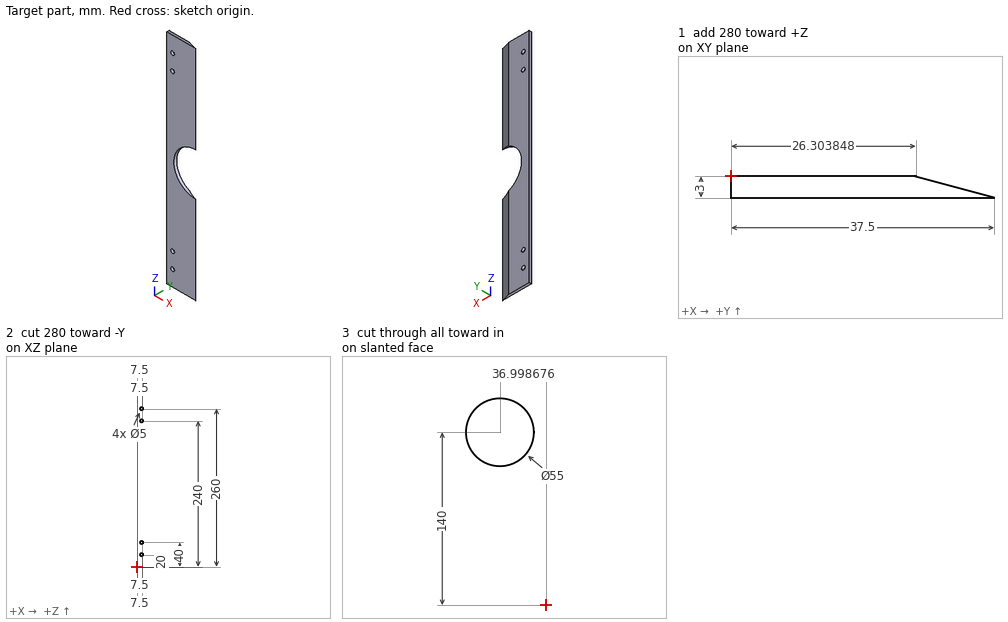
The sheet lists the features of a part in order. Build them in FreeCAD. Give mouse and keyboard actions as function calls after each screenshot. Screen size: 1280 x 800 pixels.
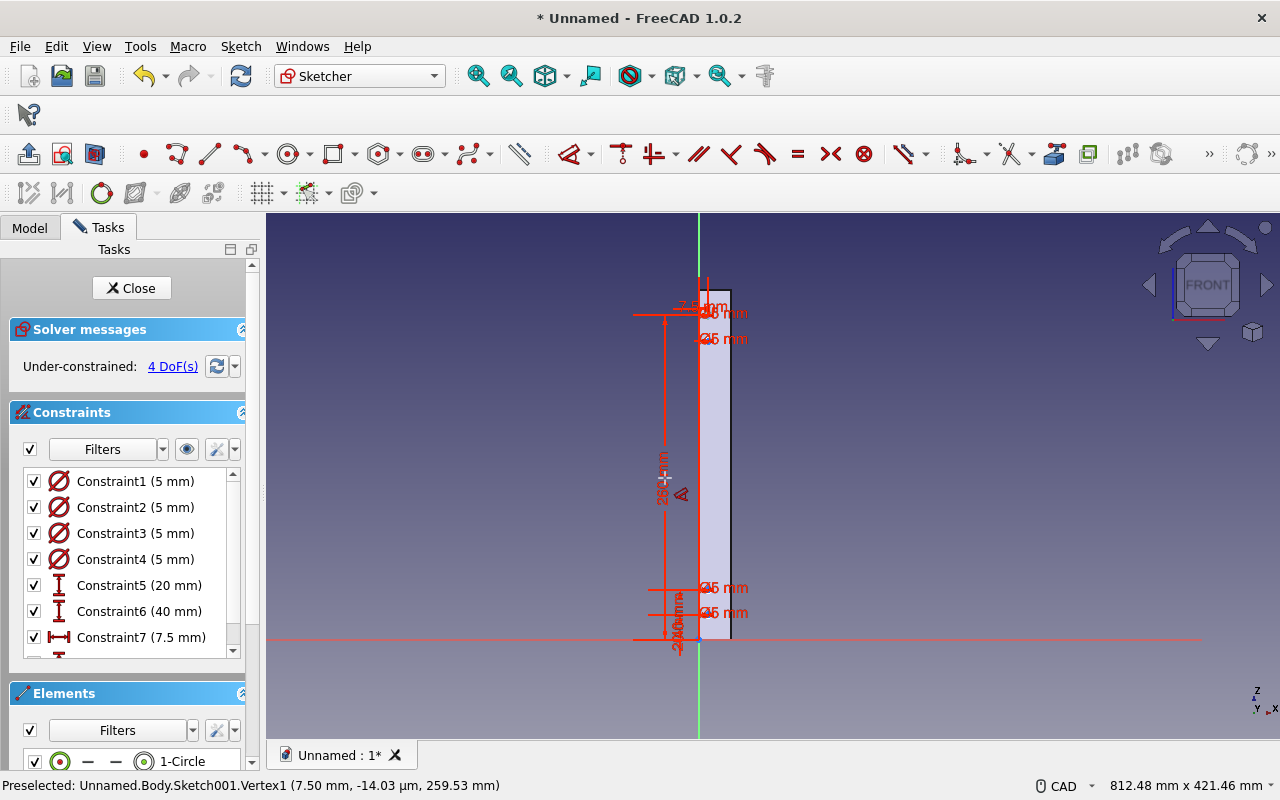
scroll(708, 341, up, 8)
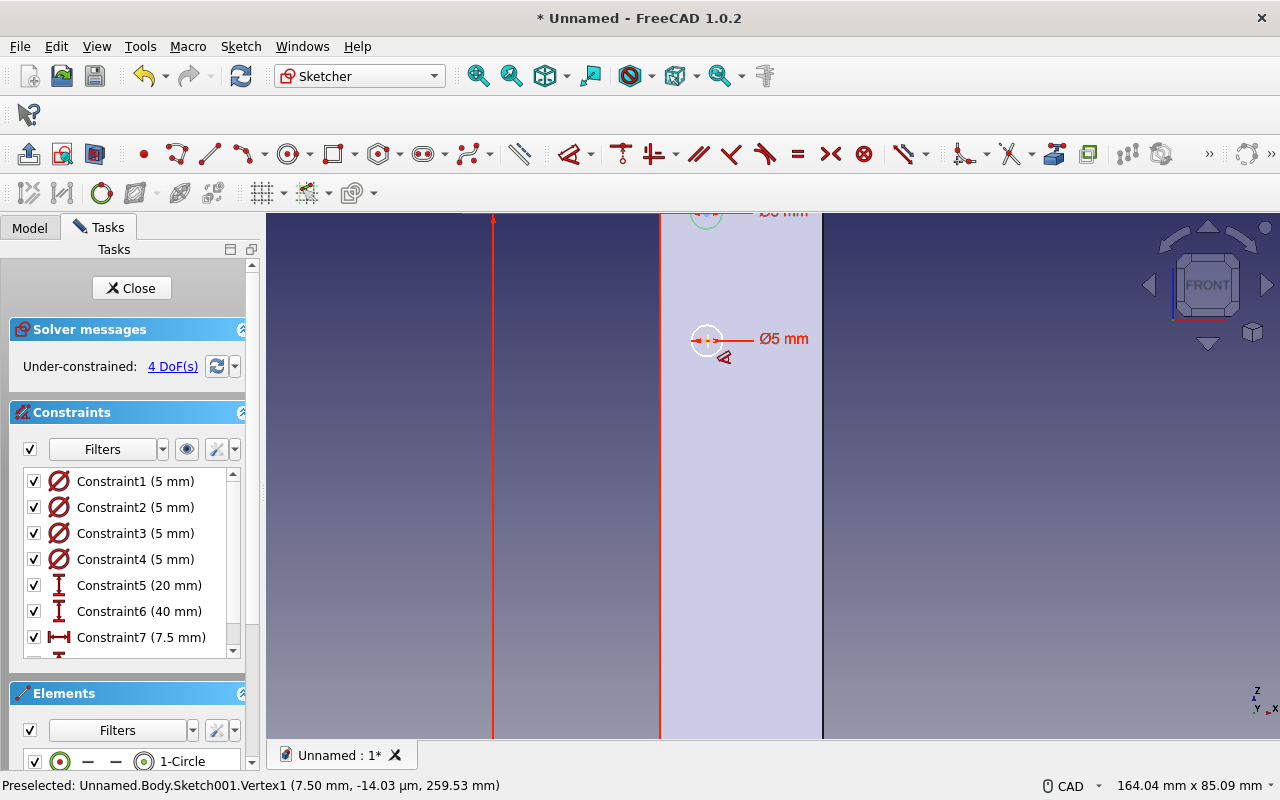
click(707, 341)
click(684, 307)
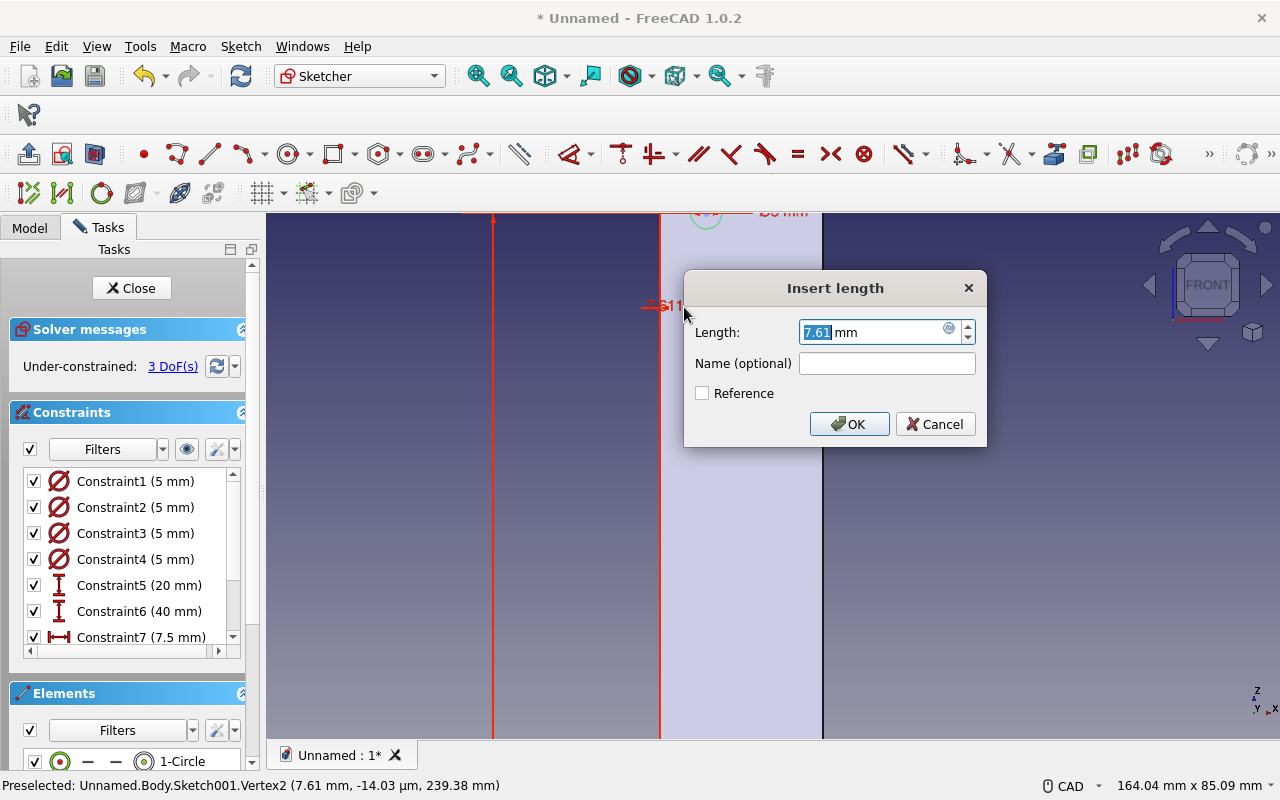
text(7.5)
key(Return)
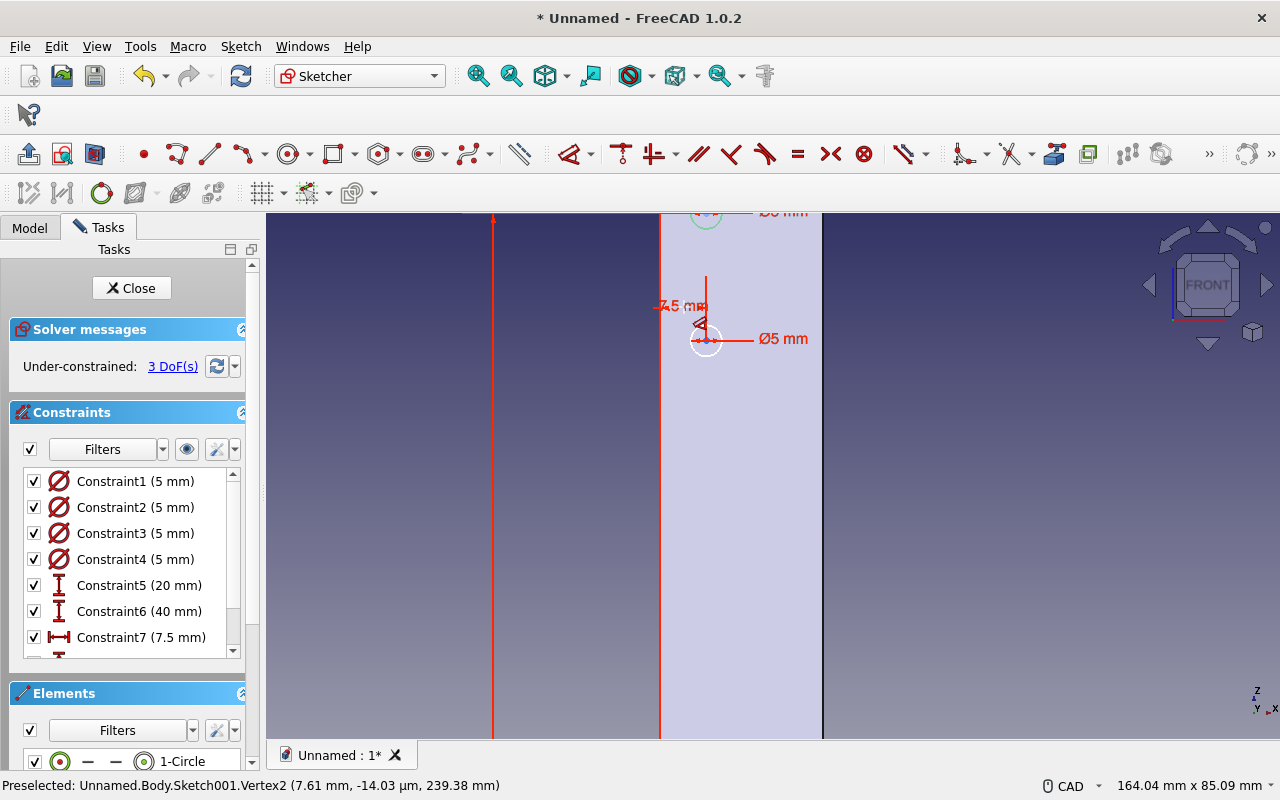
scroll(708, 341, down, 8)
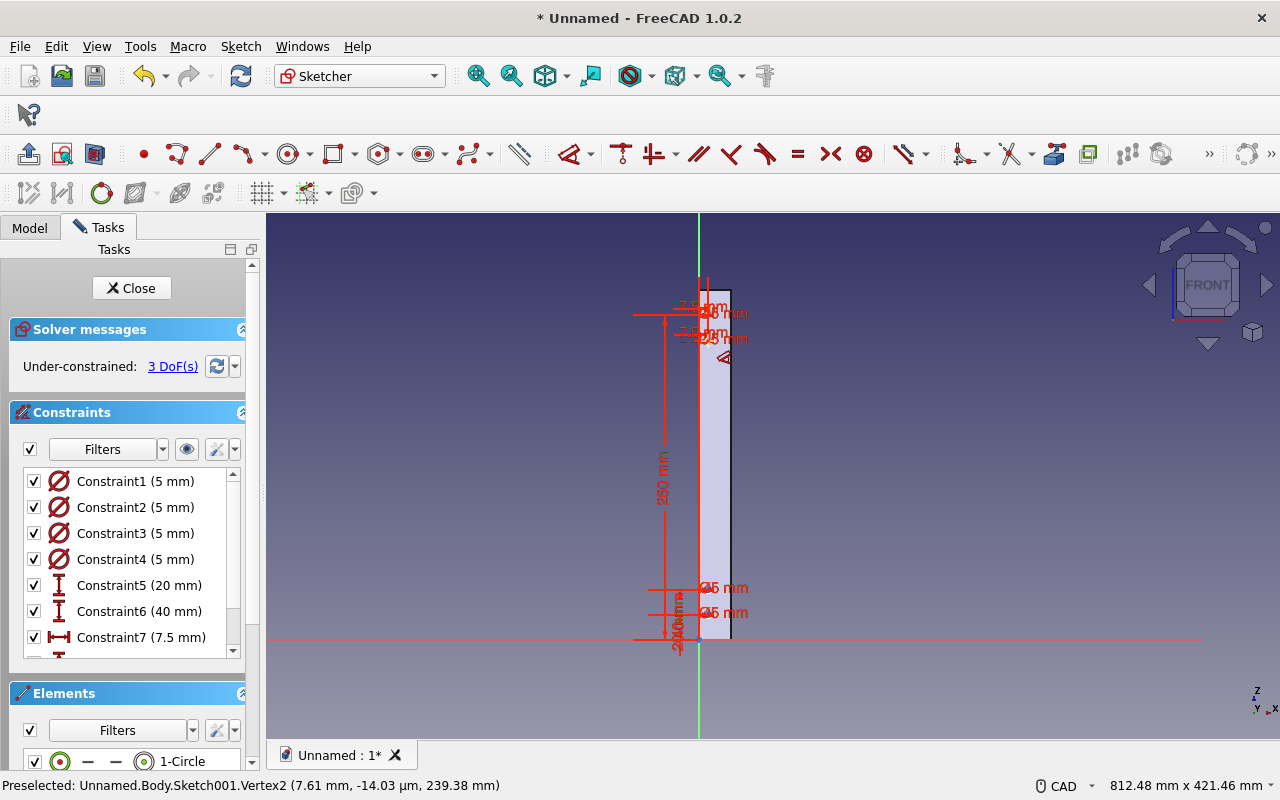
click(708, 341)
click(665, 422)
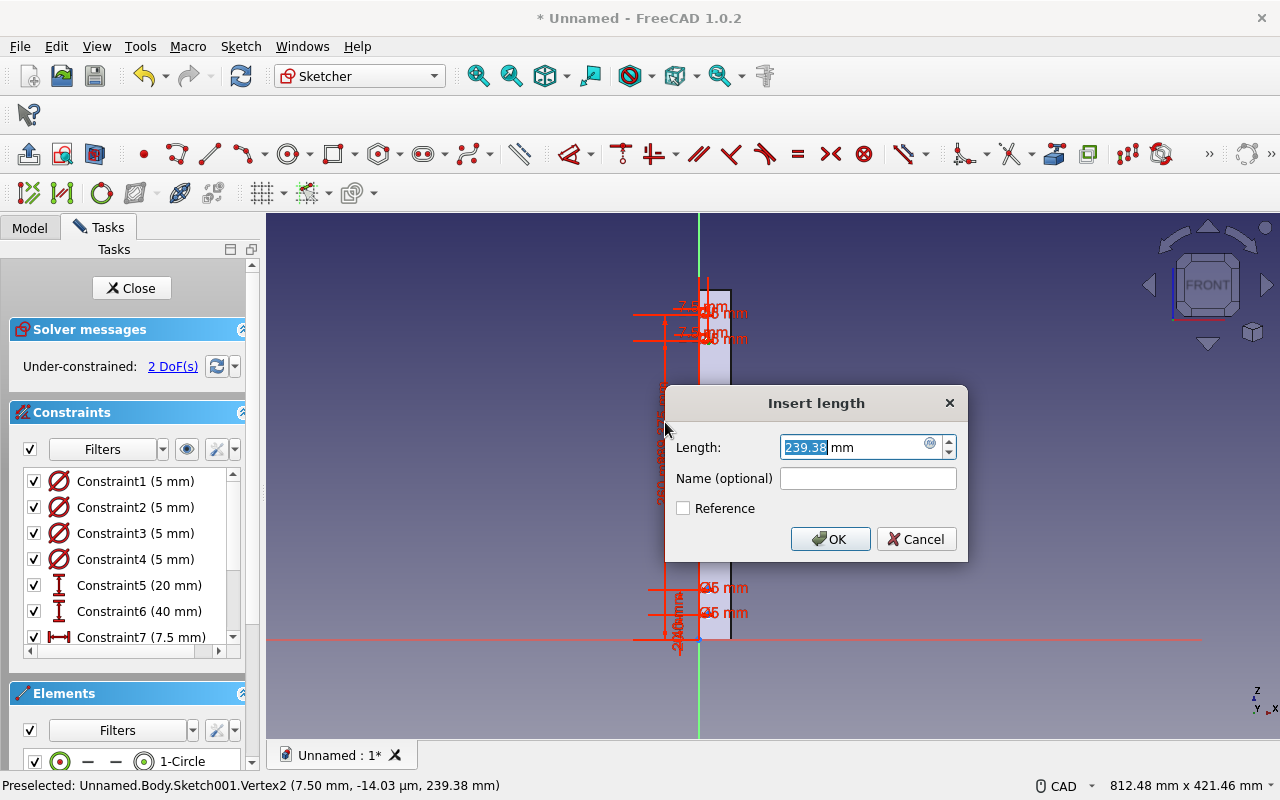
text(240)
key(Return)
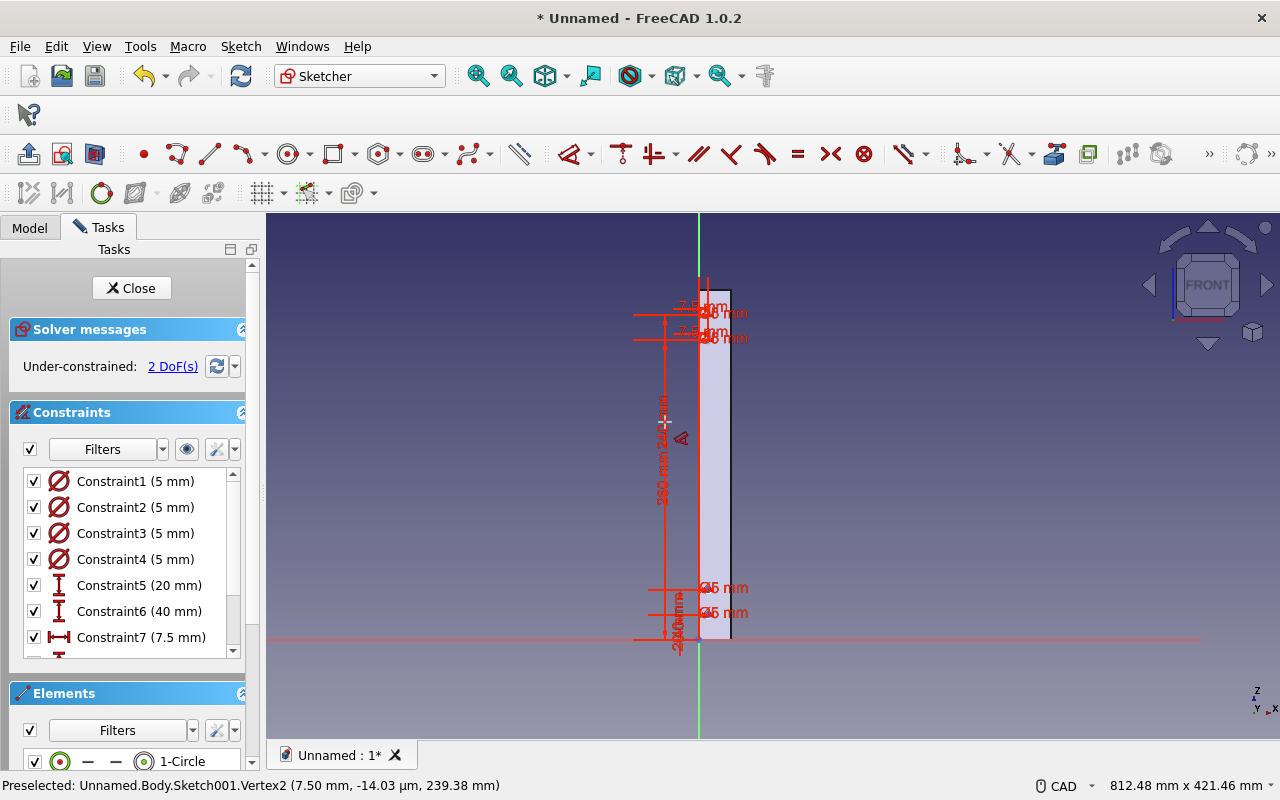
scroll(708, 615, up, 8)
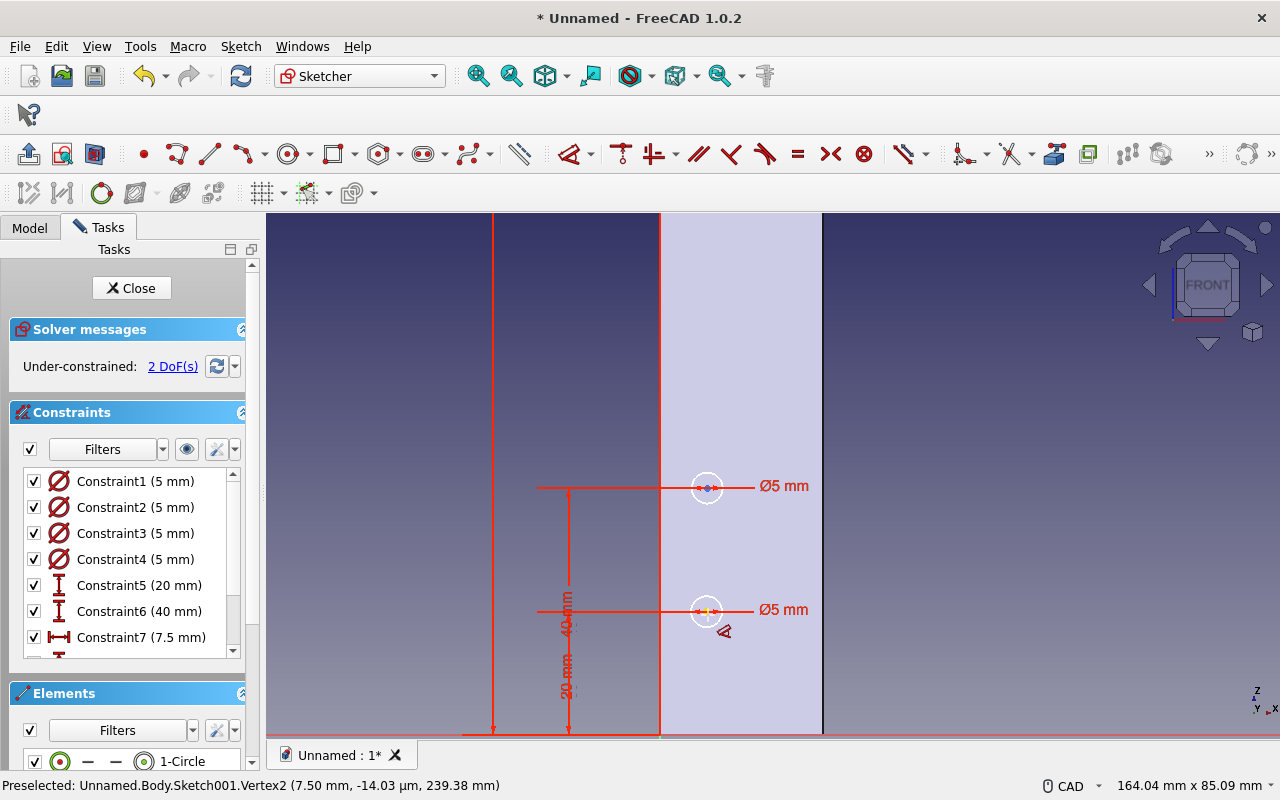
click(707, 612)
click(683, 578)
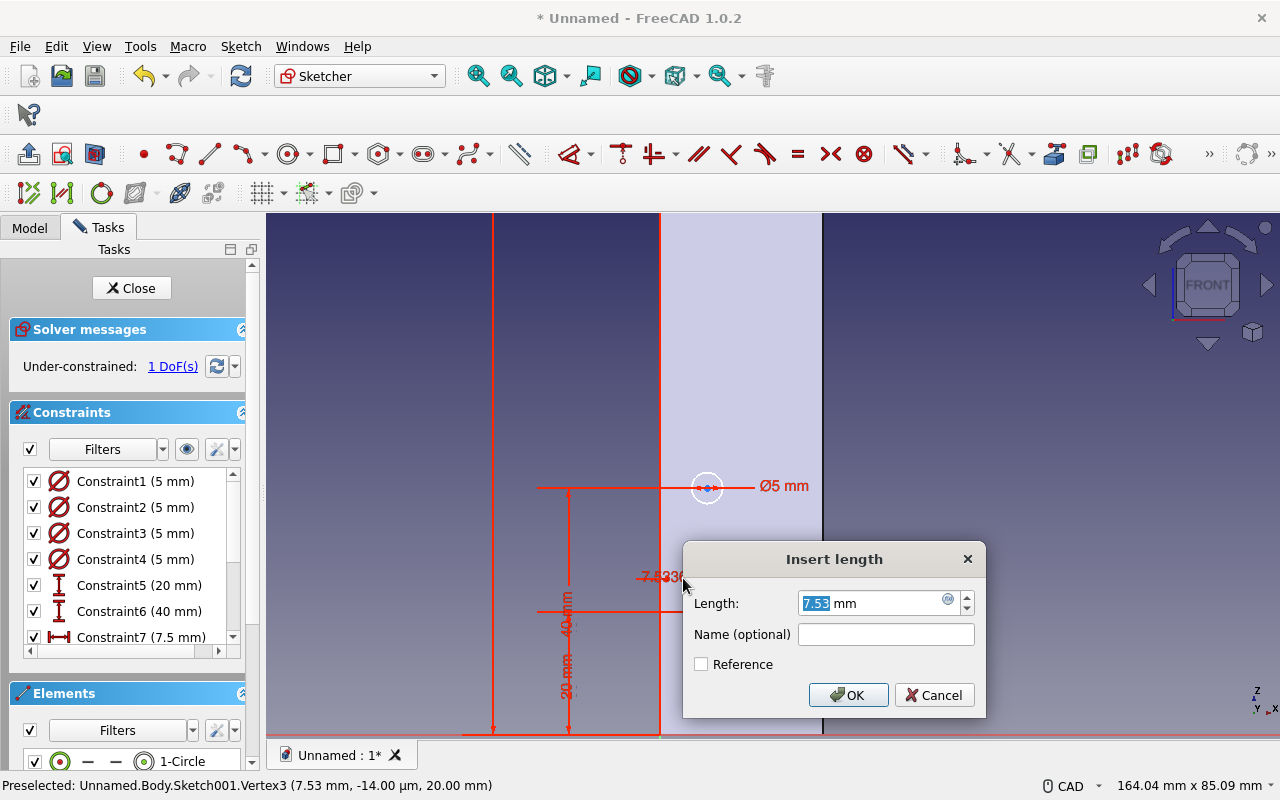
text(7.5)
key(Return)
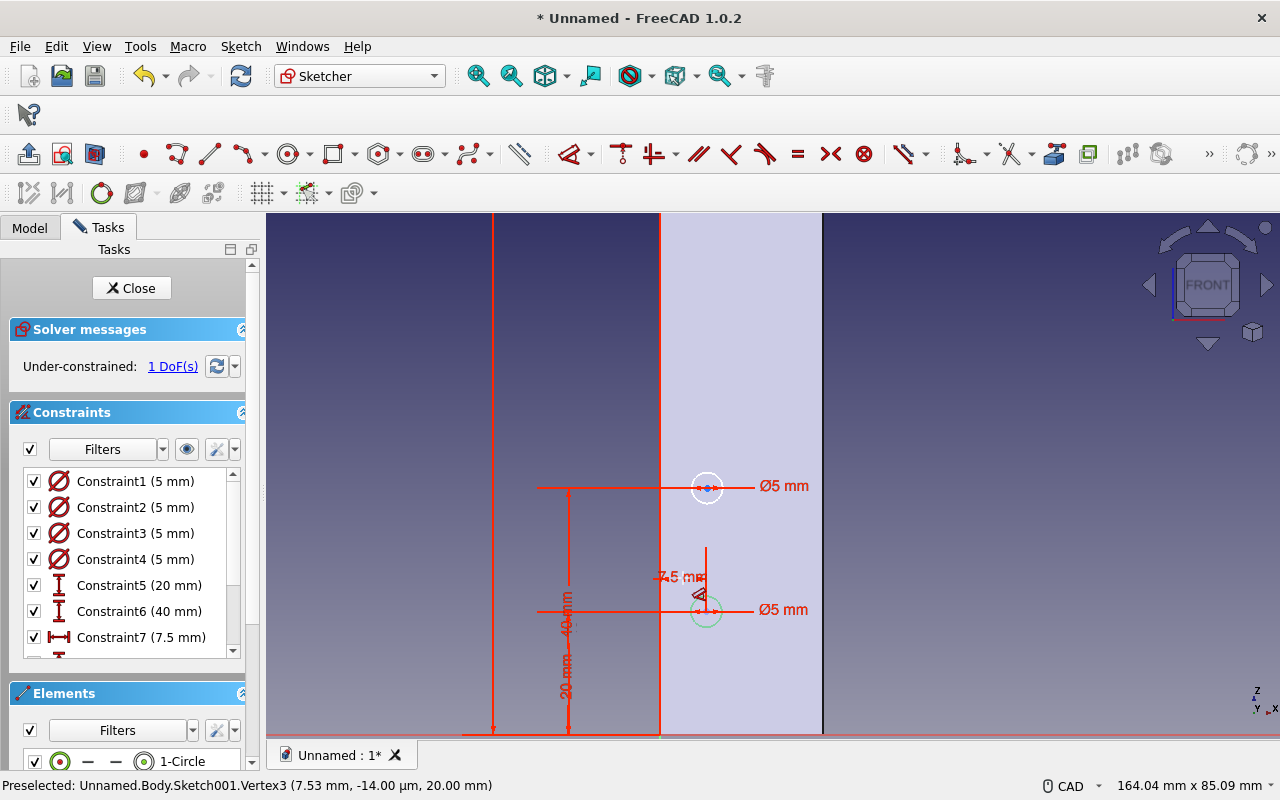
click(707, 488)
click(684, 454)